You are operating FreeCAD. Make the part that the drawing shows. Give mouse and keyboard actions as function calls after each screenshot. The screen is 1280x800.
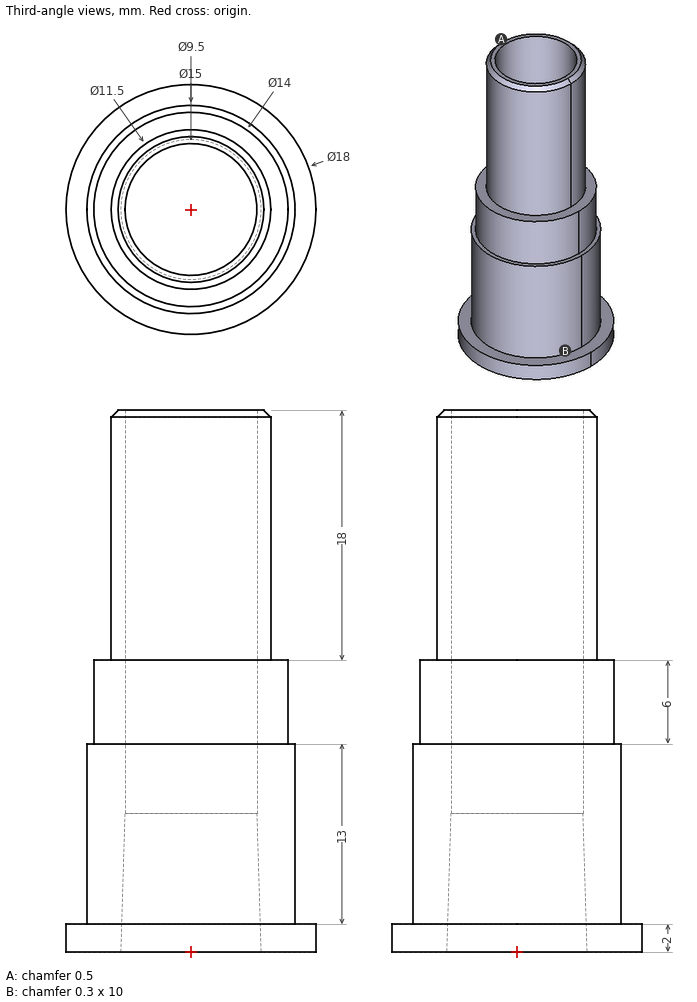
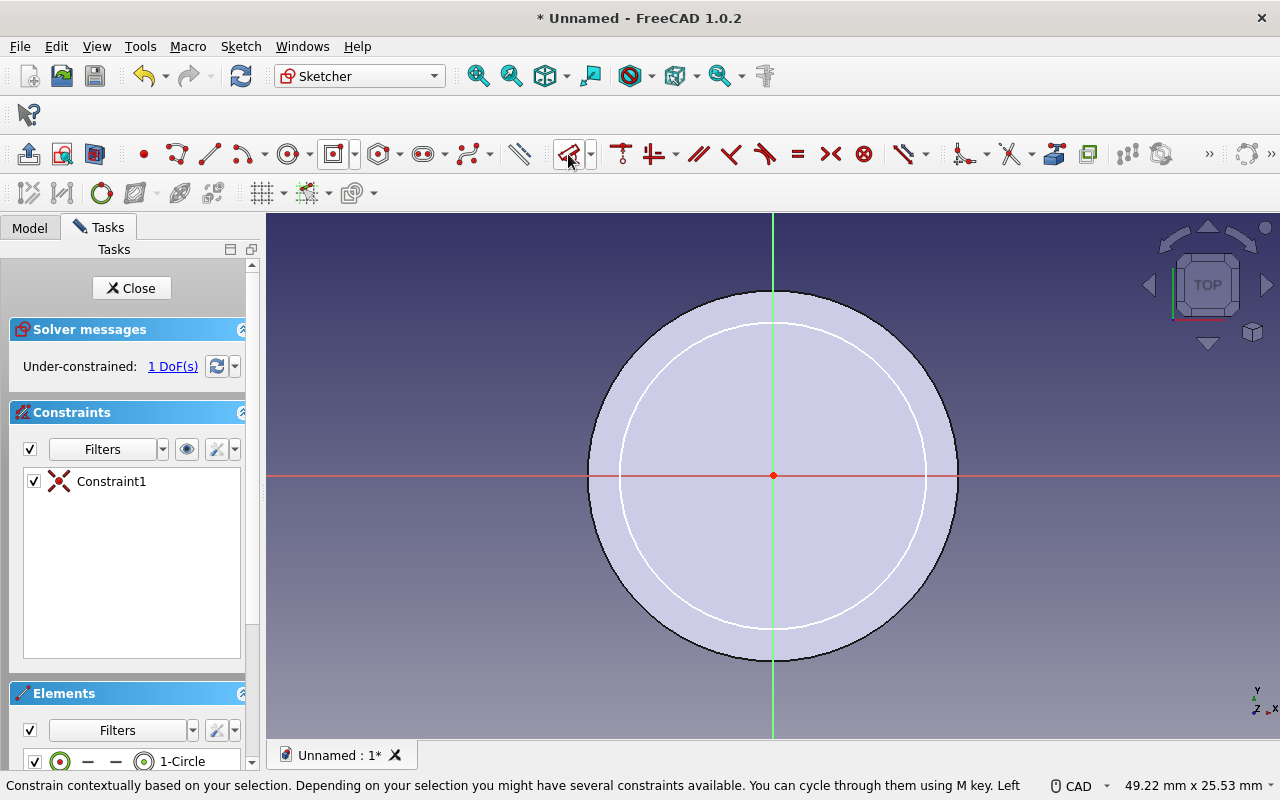
click(881, 367)
click(904, 344)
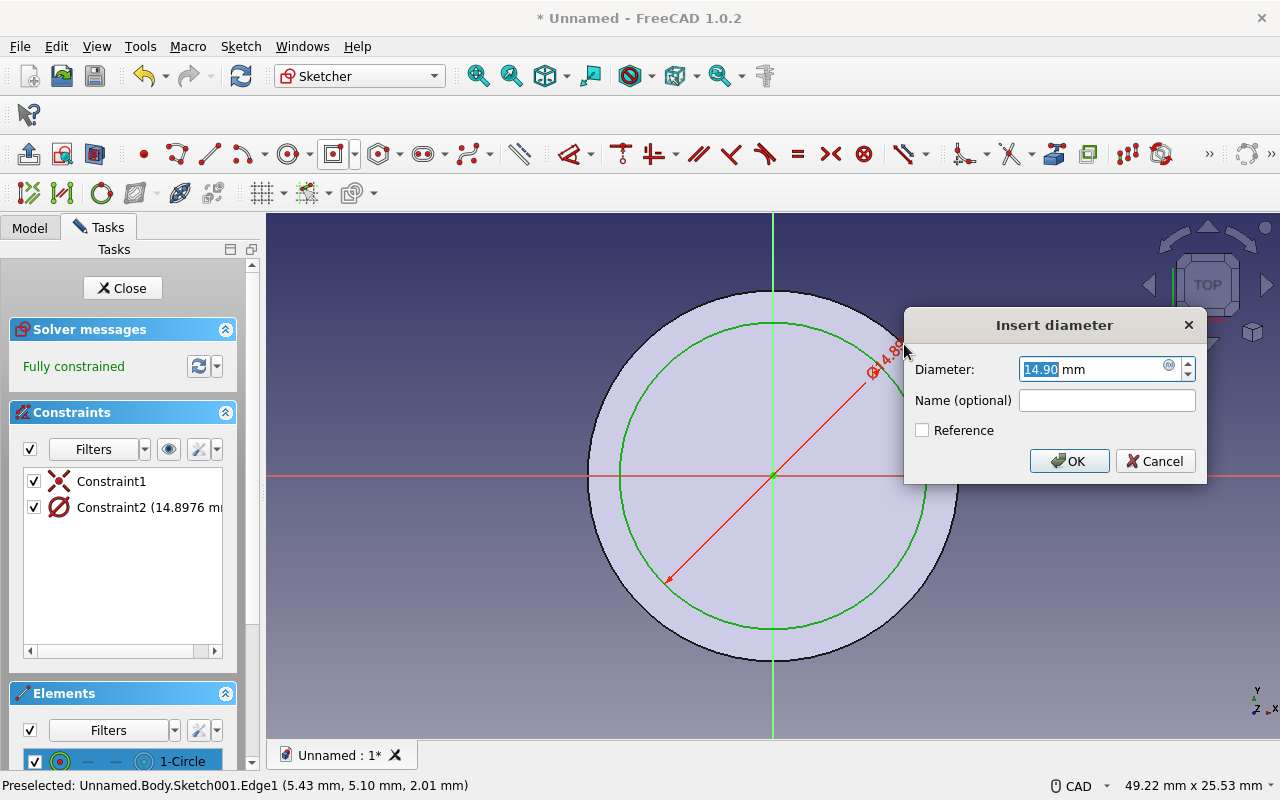
text(15)
key(Return)
key(Escape)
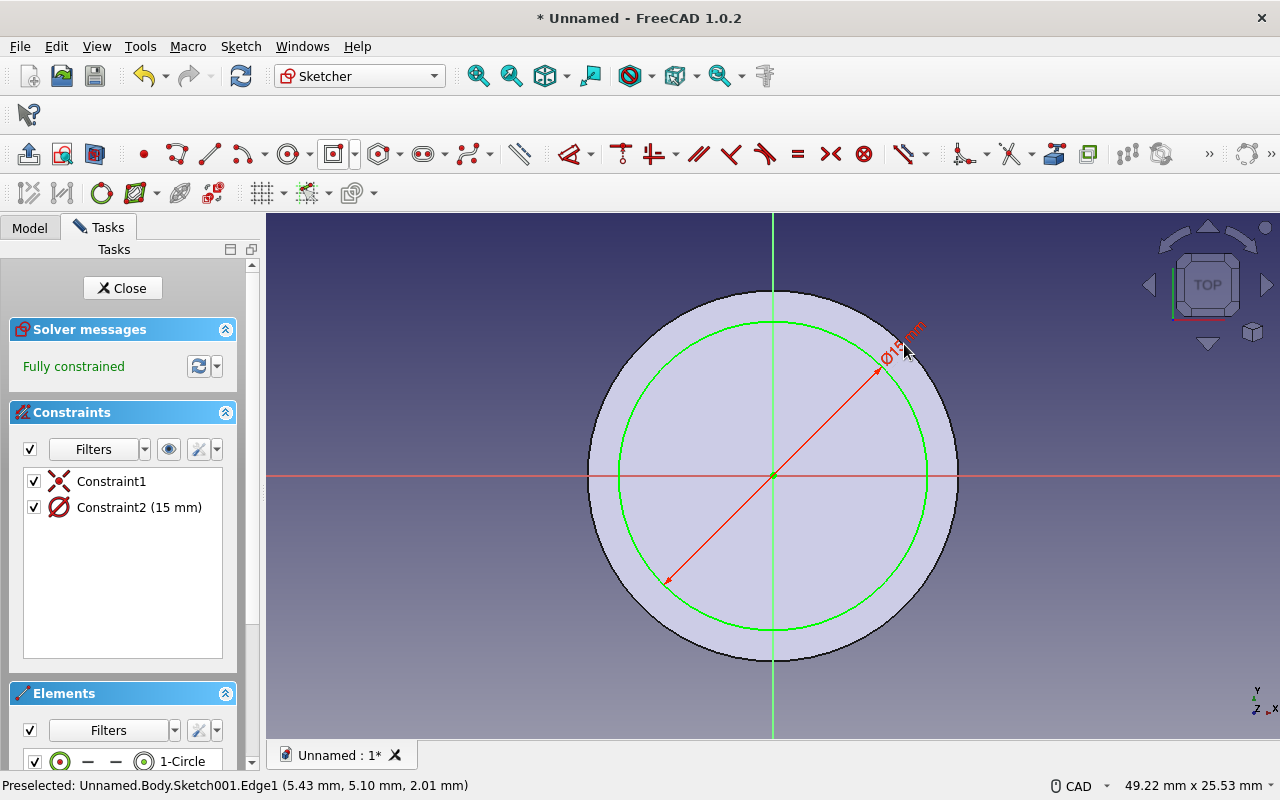
click(123, 288)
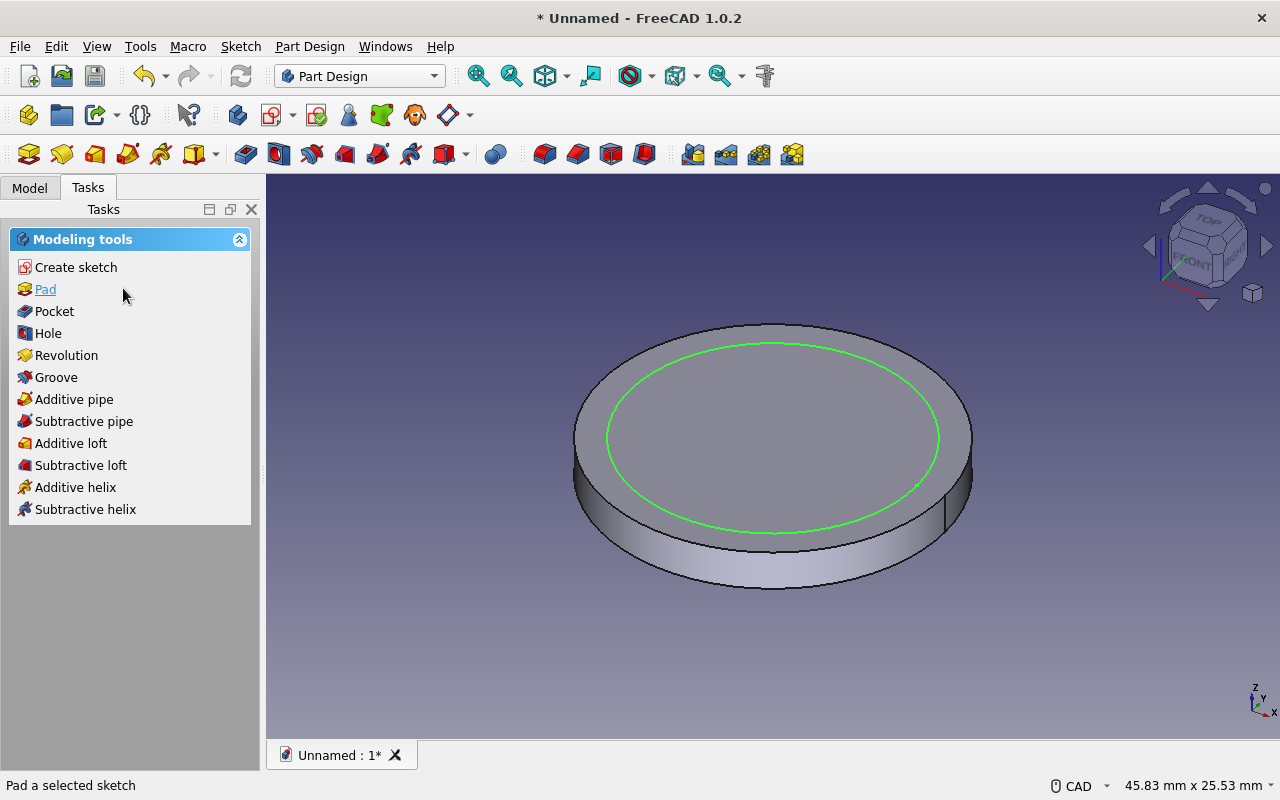
click(29, 154)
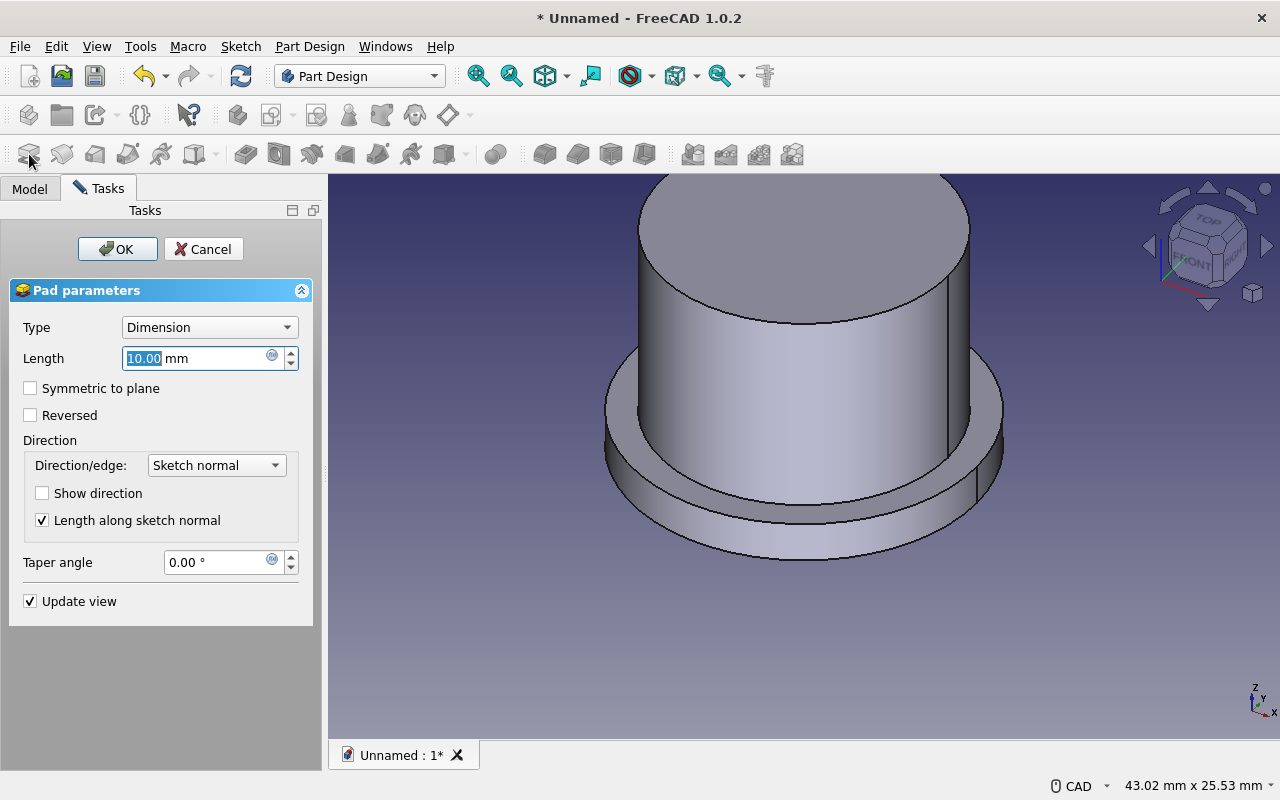
text(13)
key(Tab)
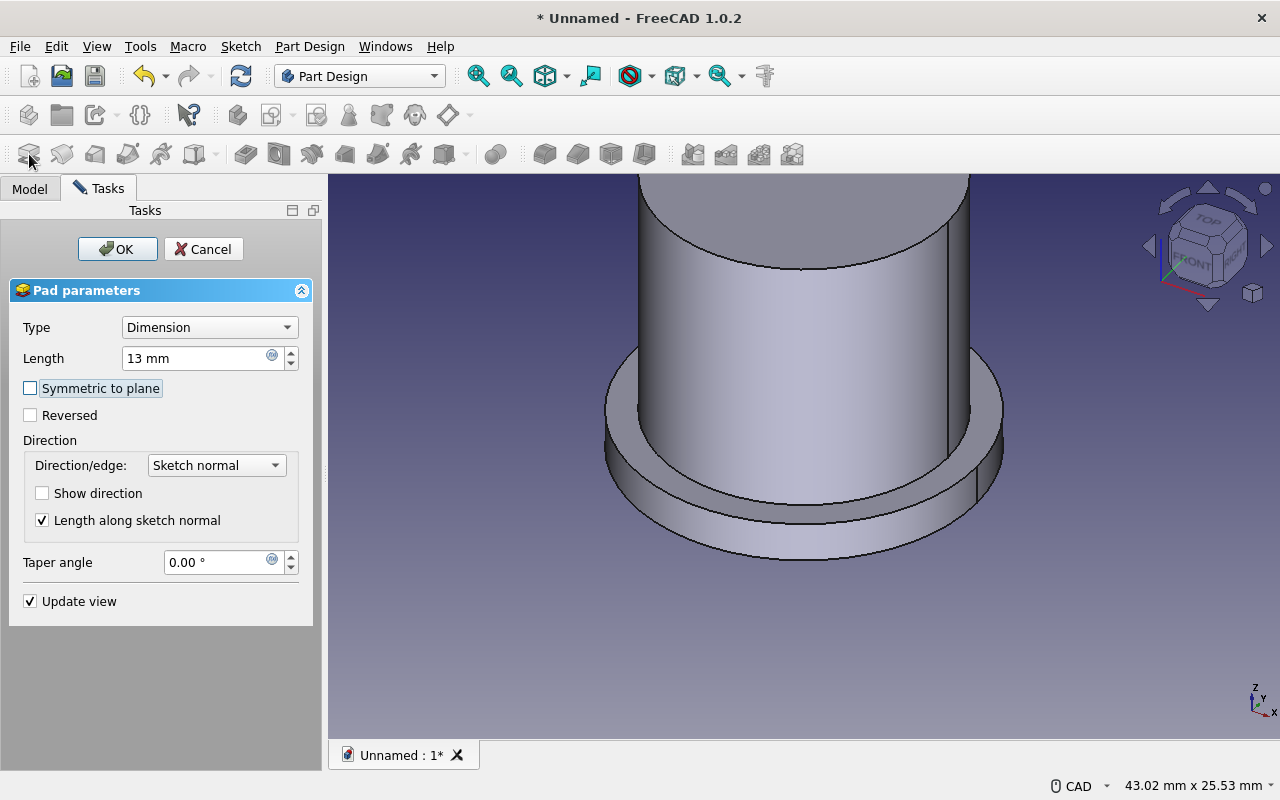
click(118, 249)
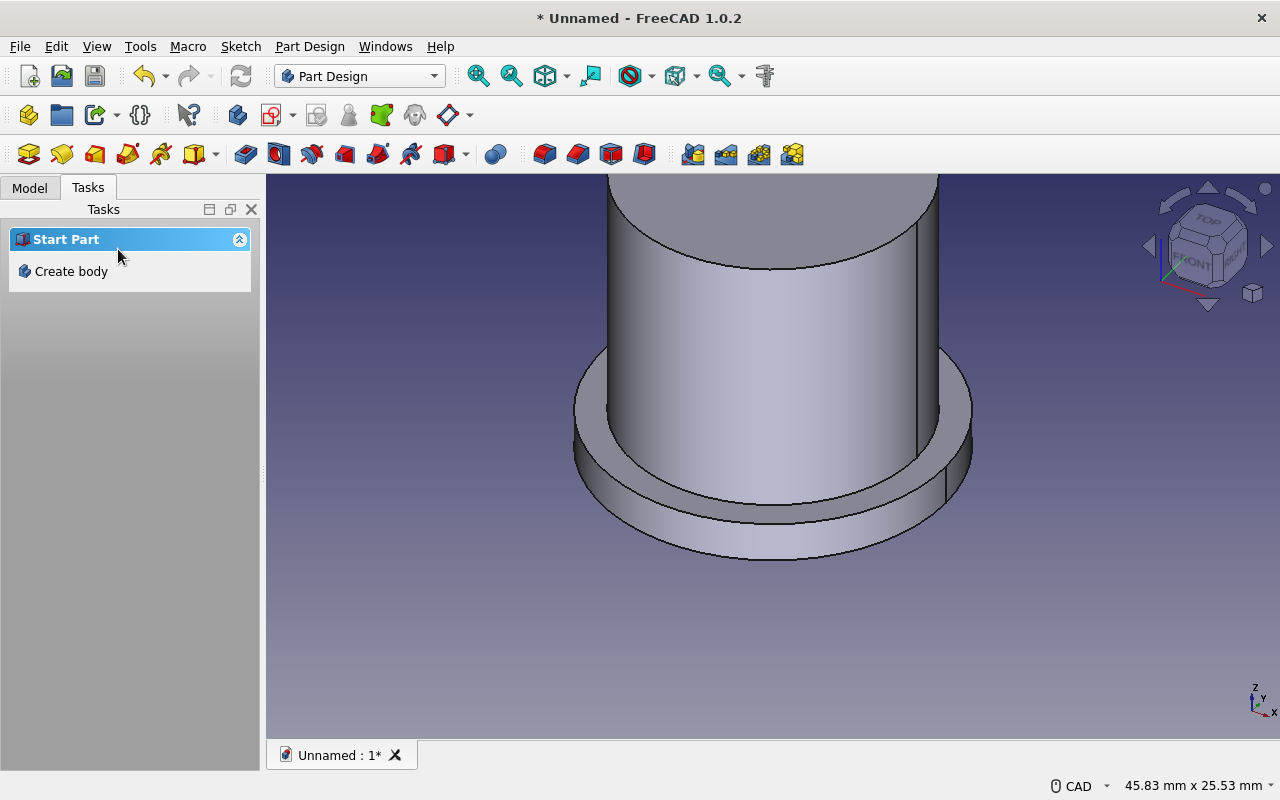
click(479, 76)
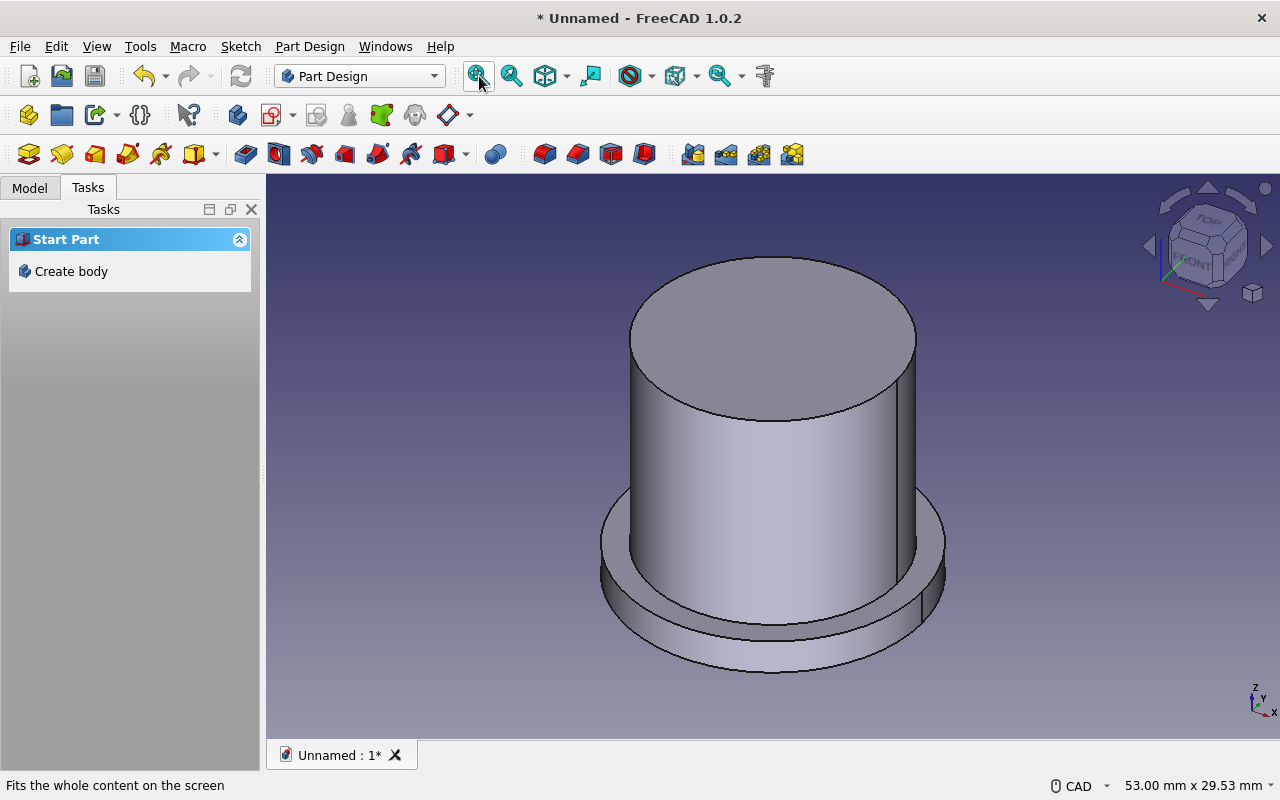
click(773, 338)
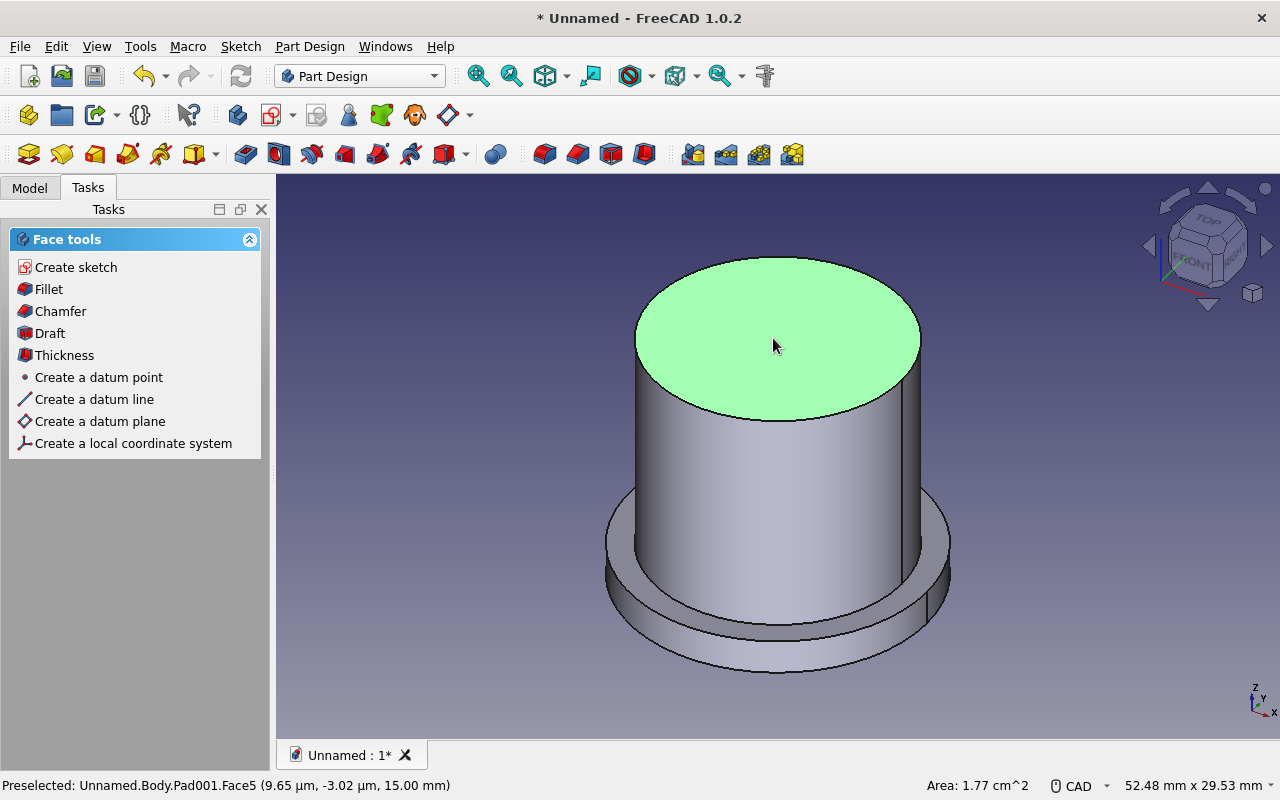
click(270, 116)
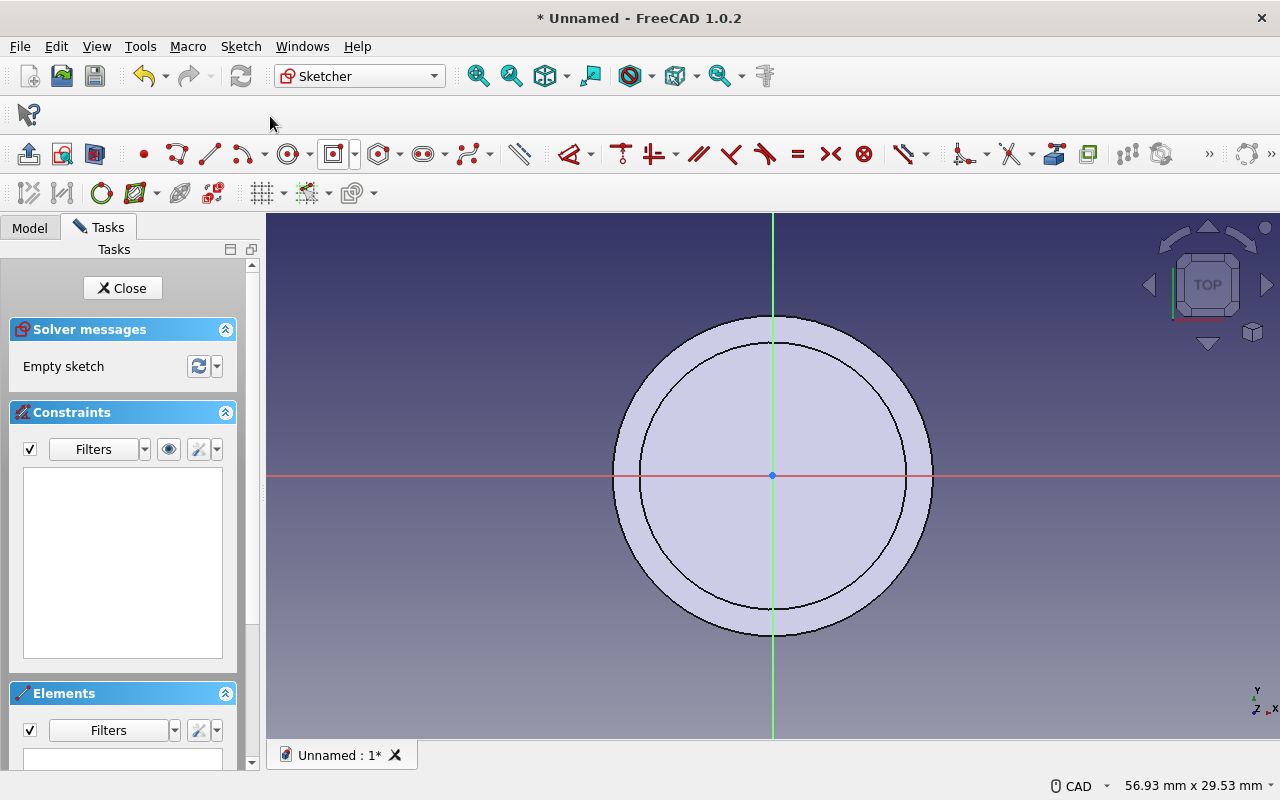
click(288, 154)